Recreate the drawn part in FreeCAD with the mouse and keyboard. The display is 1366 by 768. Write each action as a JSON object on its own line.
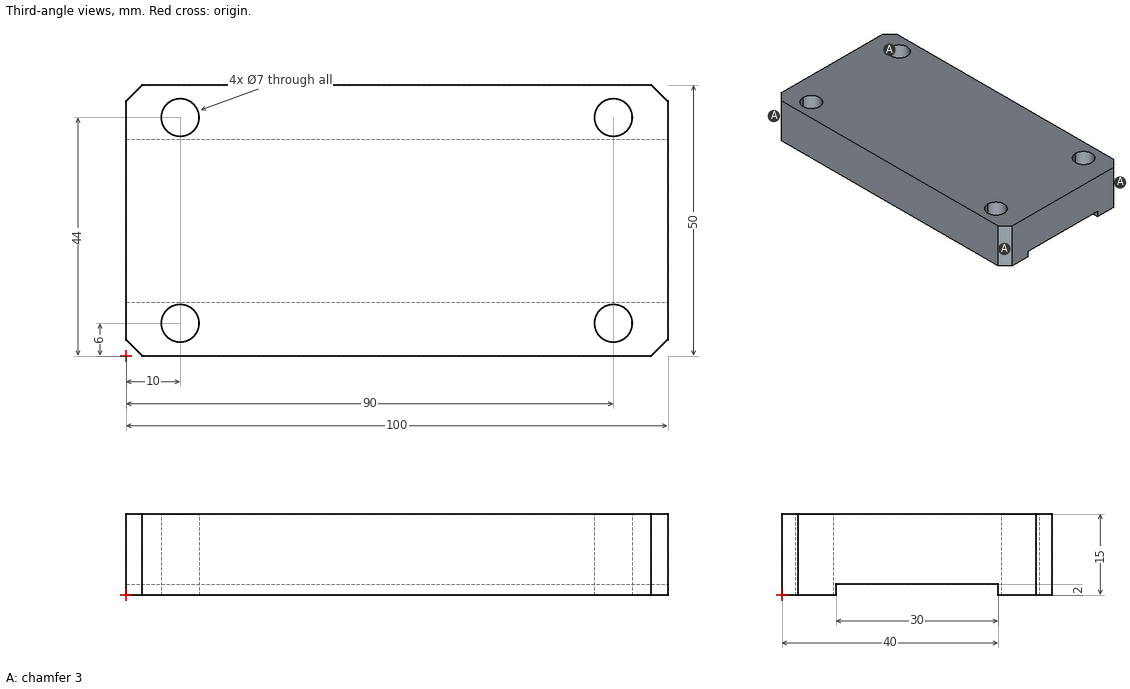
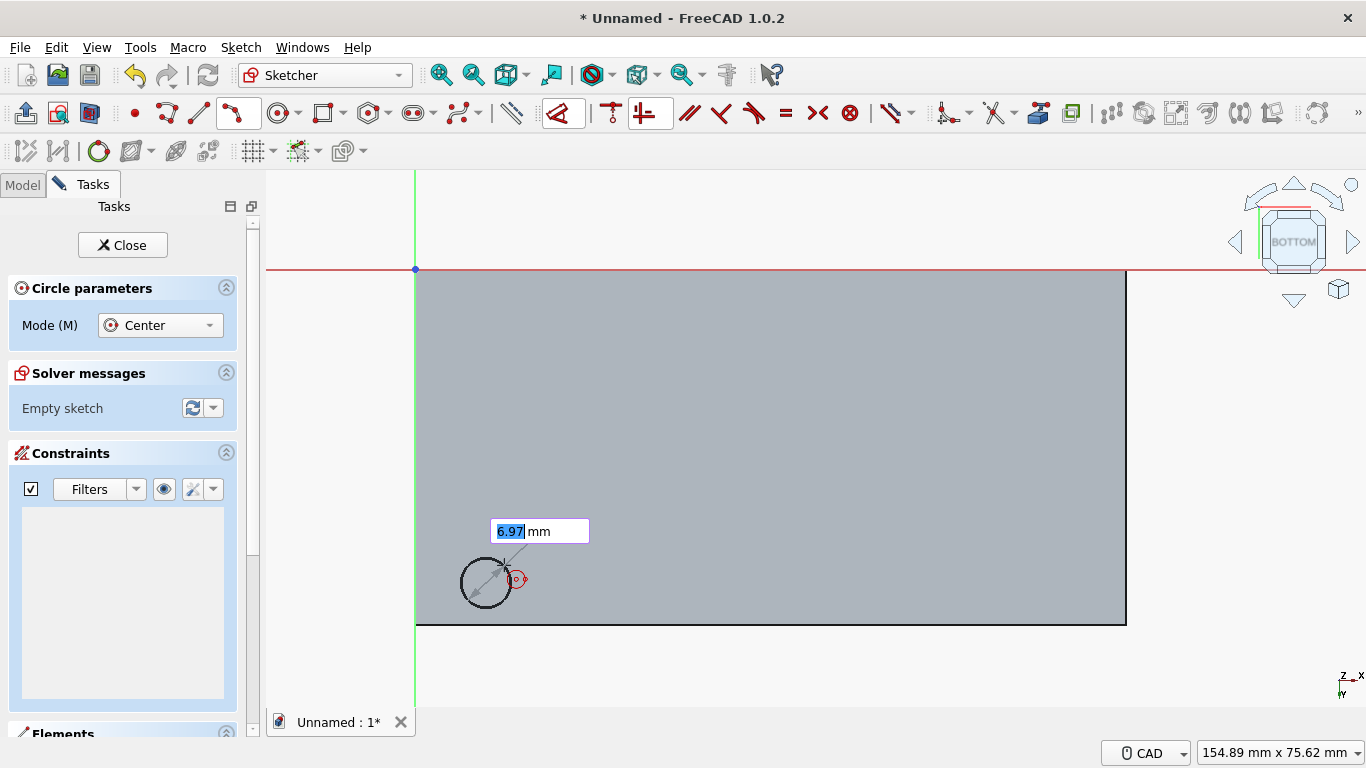
{"action": "type", "text": "7"}
{"action": "key", "text": "Return"}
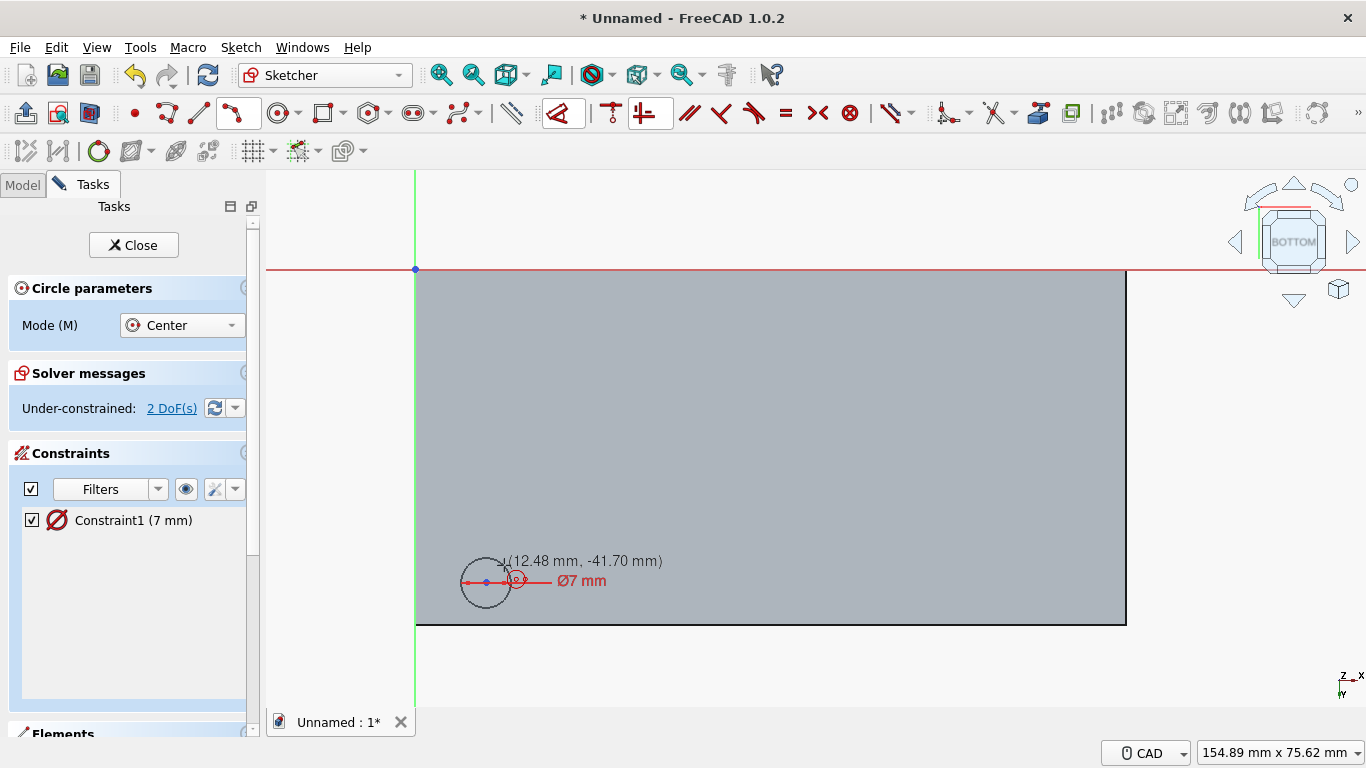
{"action": "left_click", "coordinate": [486, 312]}
{"action": "mouse_move", "coordinate": [504, 295]}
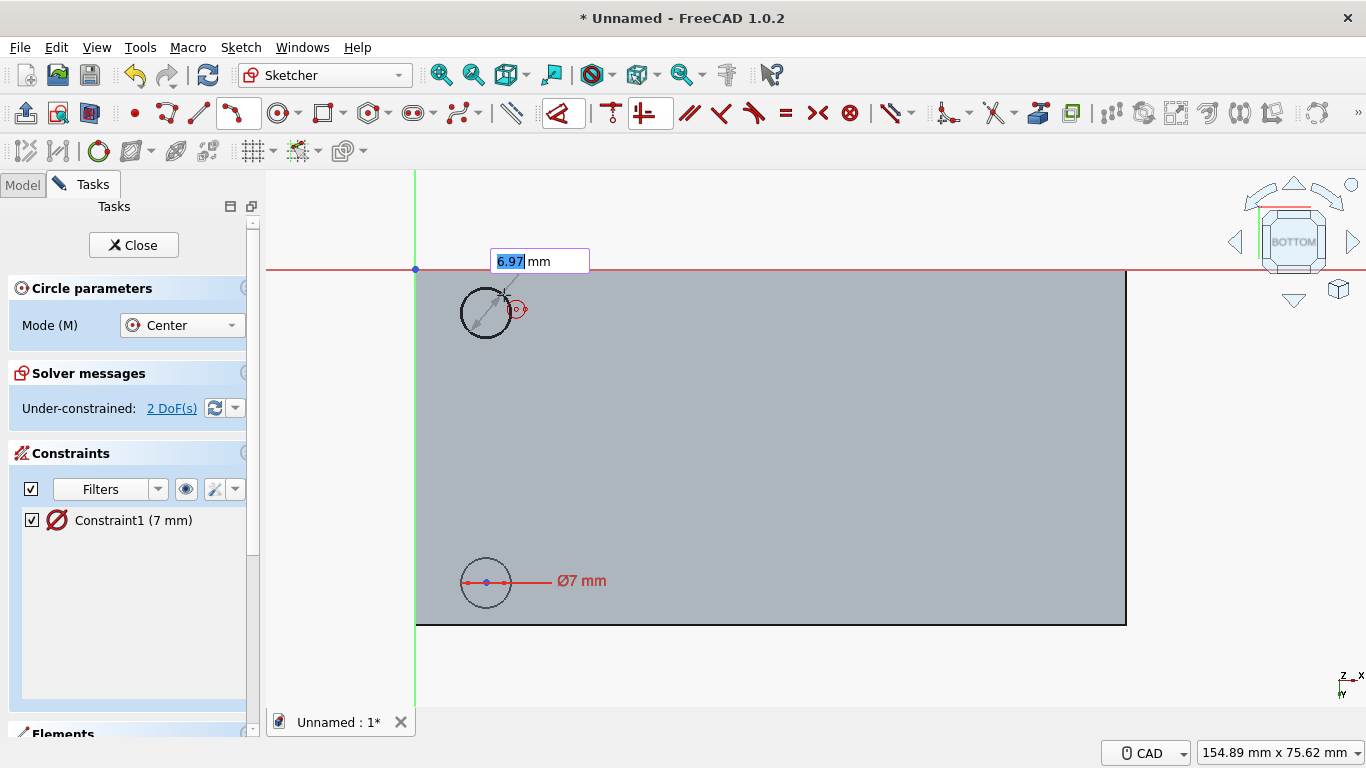
{"action": "type", "text": "7"}
{"action": "key", "text": "Return"}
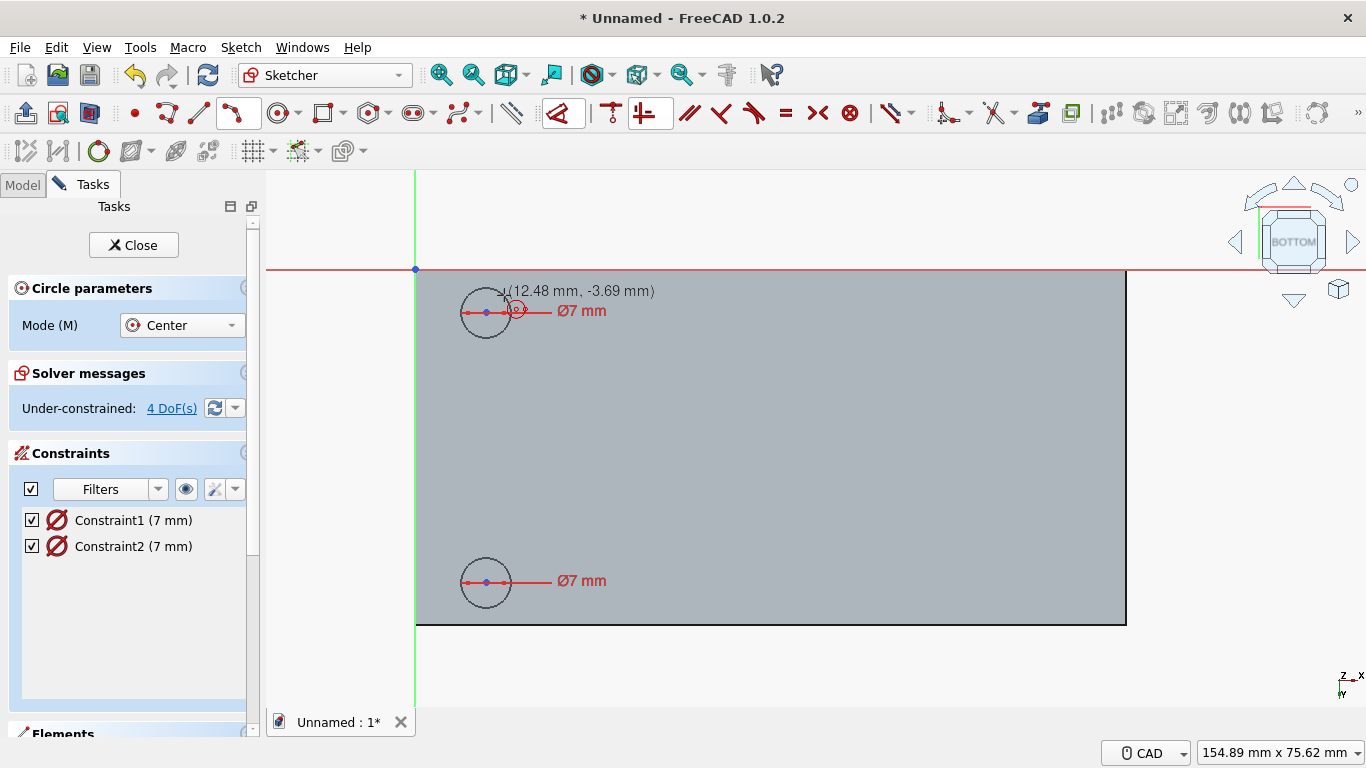
{"action": "left_click", "coordinate": [1055, 582]}
{"action": "mouse_move", "coordinate": [1072, 565]}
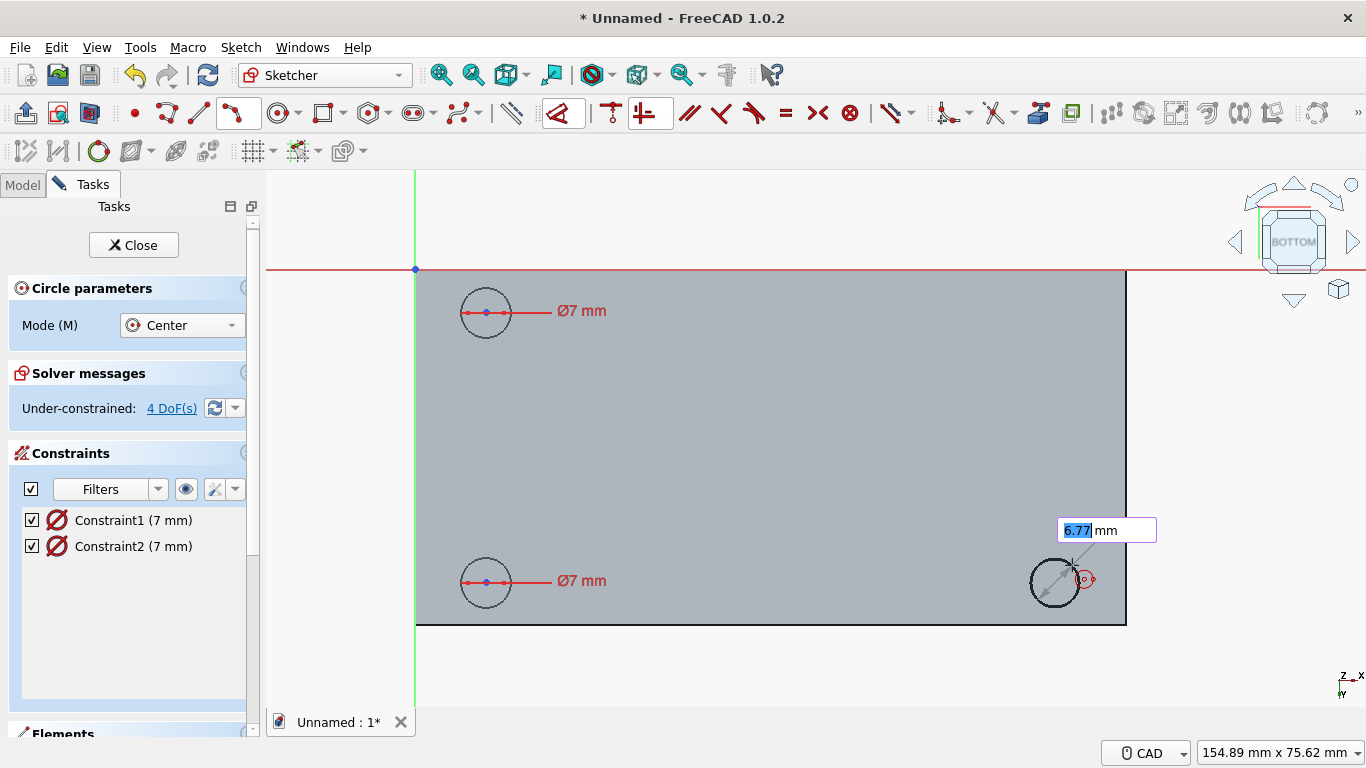
{"action": "type", "text": "7"}
{"action": "key", "text": "Return"}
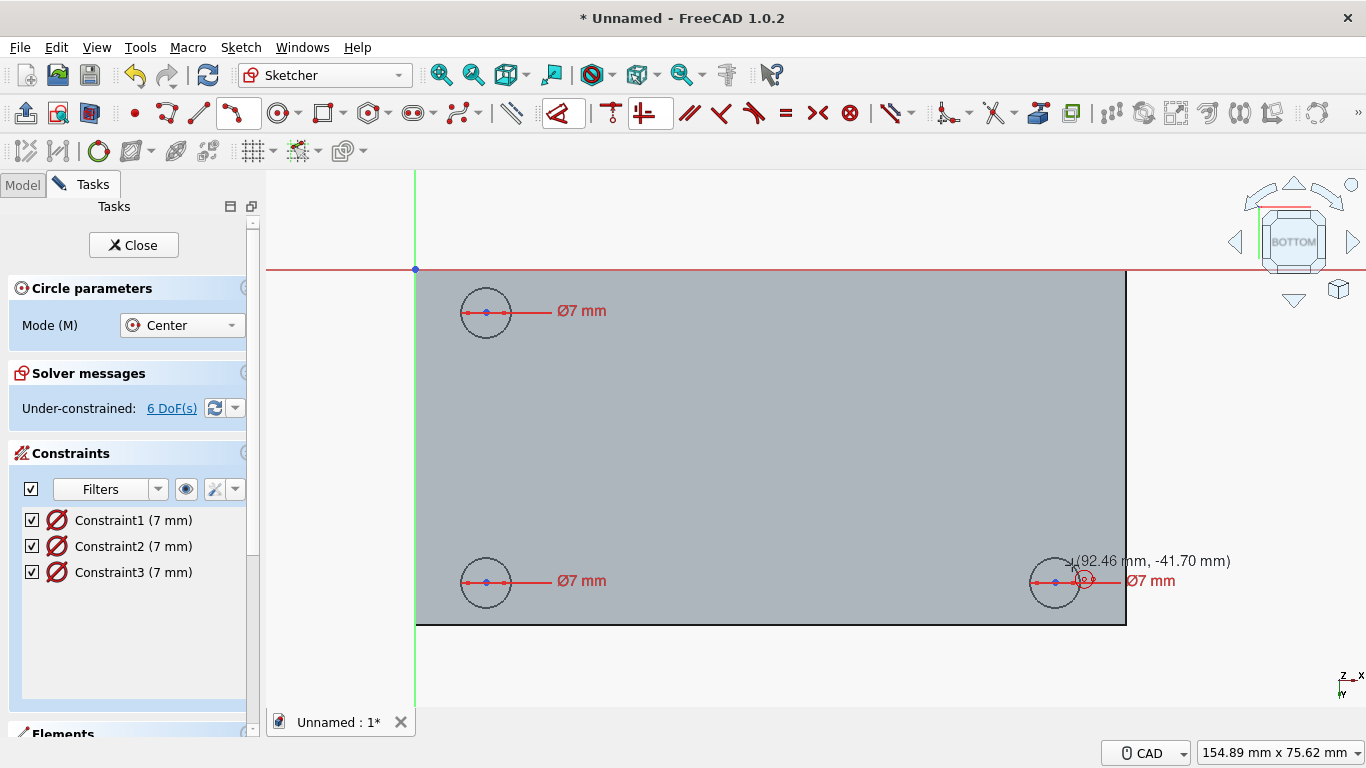
{"action": "left_click", "coordinate": [1055, 312]}
{"action": "mouse_move", "coordinate": [1072, 295]}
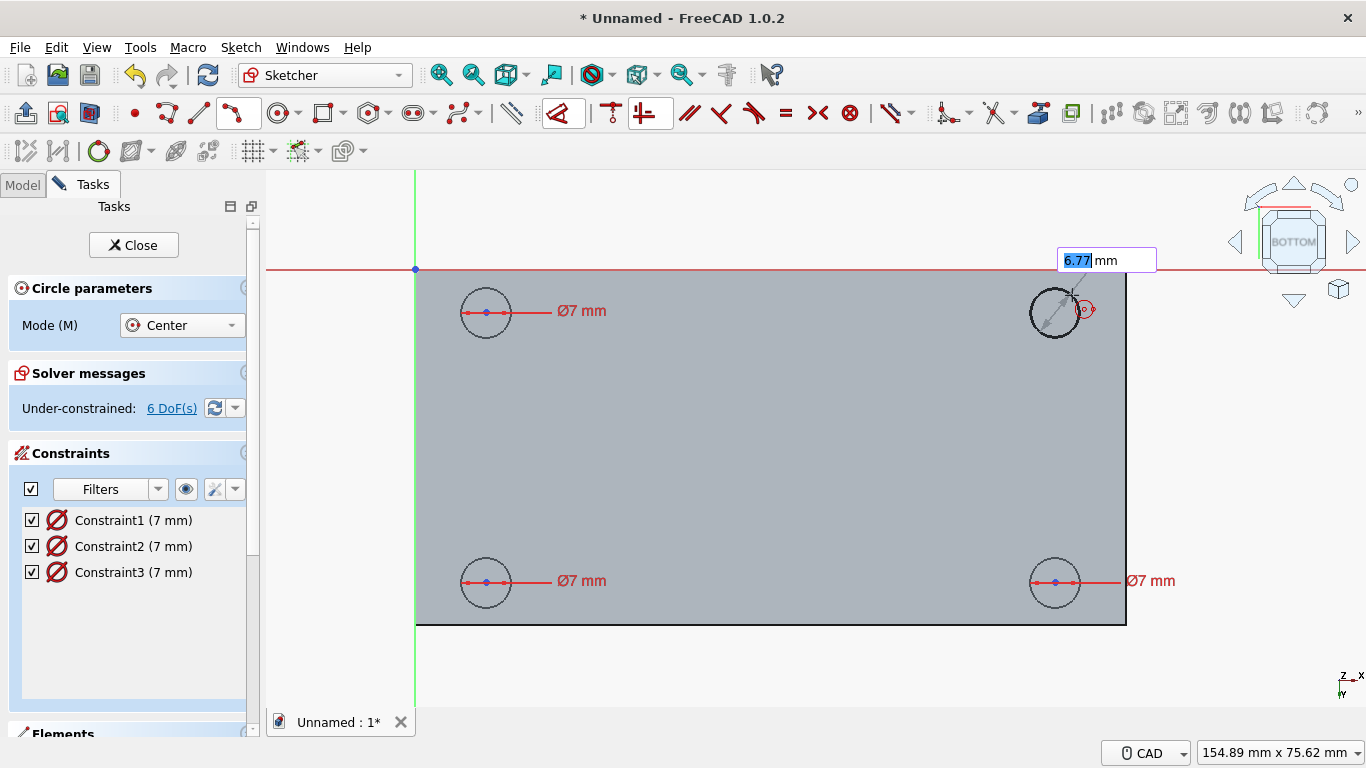
{"action": "type", "text": "7"}
{"action": "key", "text": "Return"}
{"action": "key", "text": "Escape"}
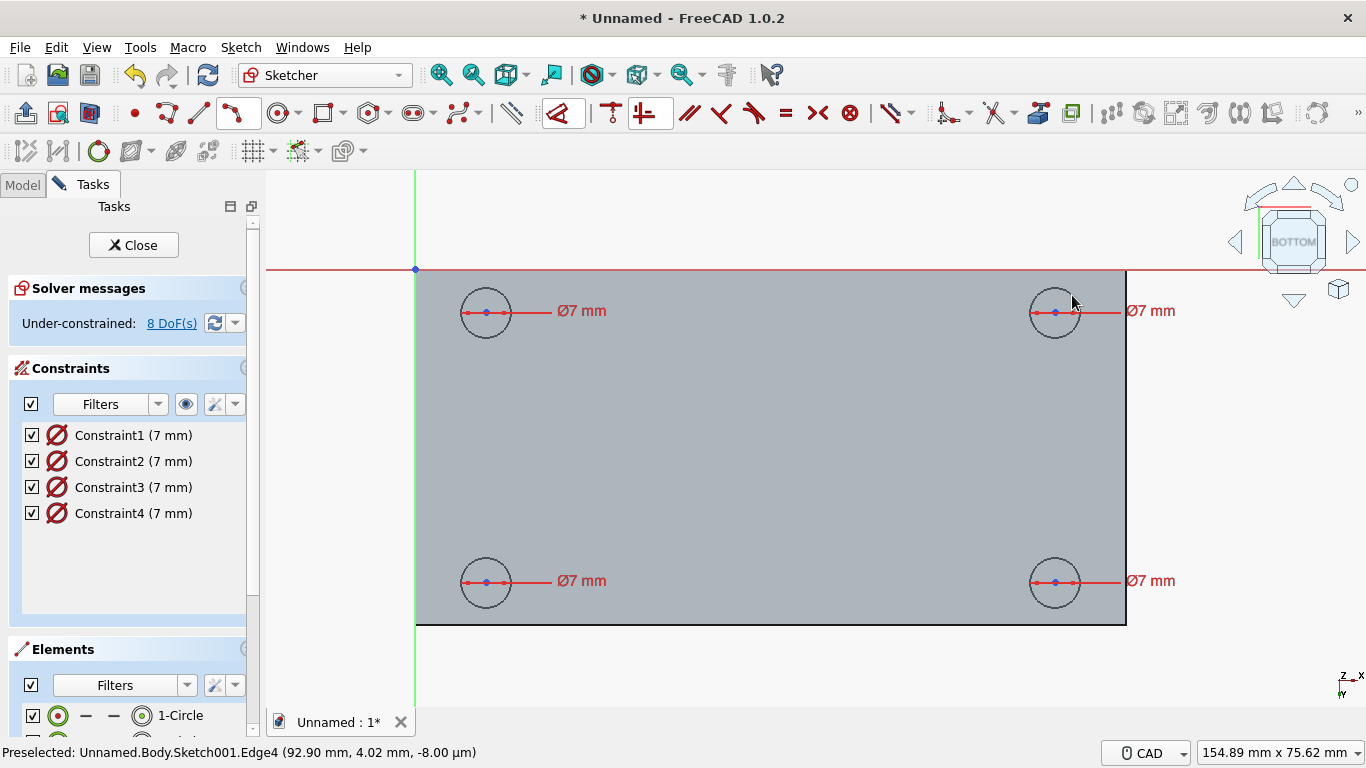
{"action": "left_click", "coordinate": [486, 583]}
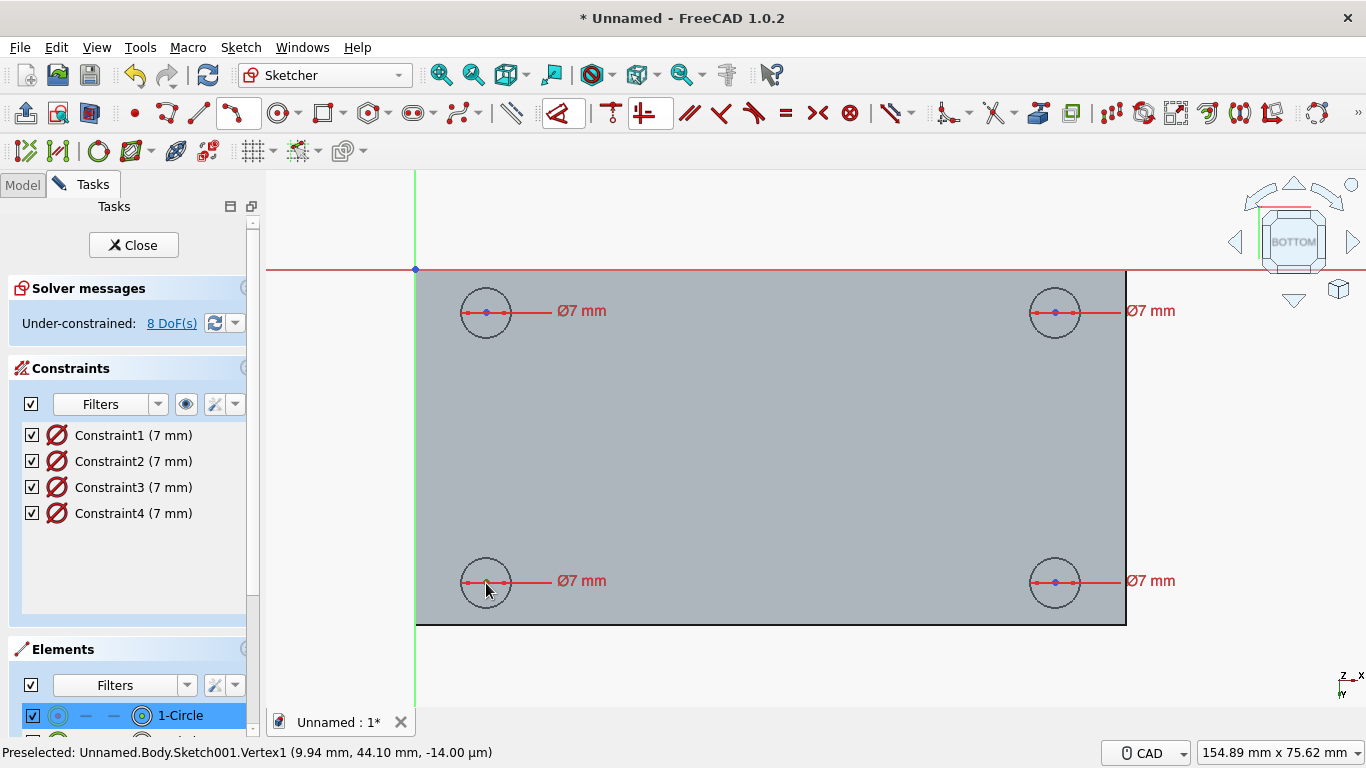
{"action": "left_click", "coordinate": [486, 313]}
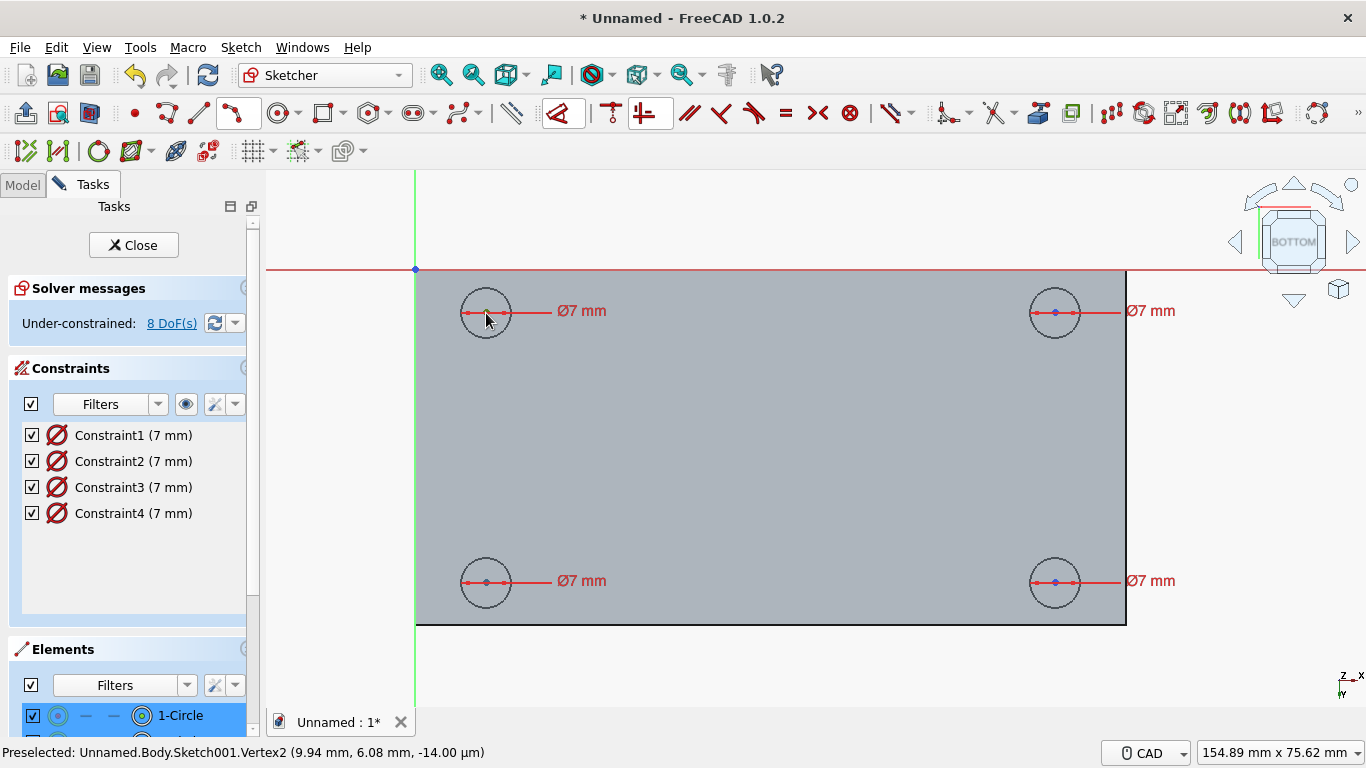
{"action": "key", "text": "v"}